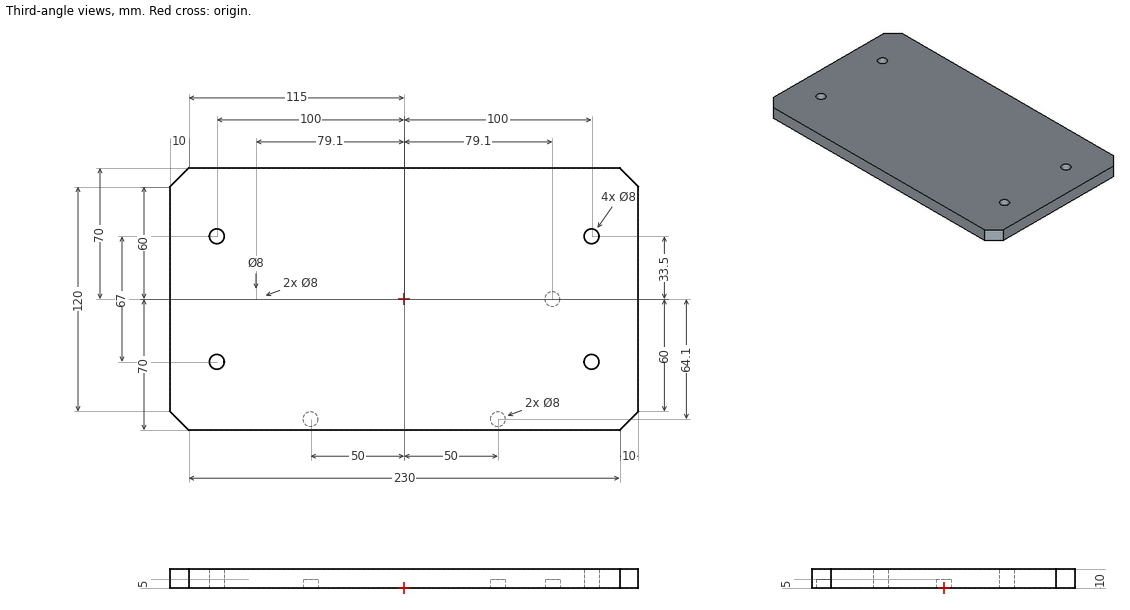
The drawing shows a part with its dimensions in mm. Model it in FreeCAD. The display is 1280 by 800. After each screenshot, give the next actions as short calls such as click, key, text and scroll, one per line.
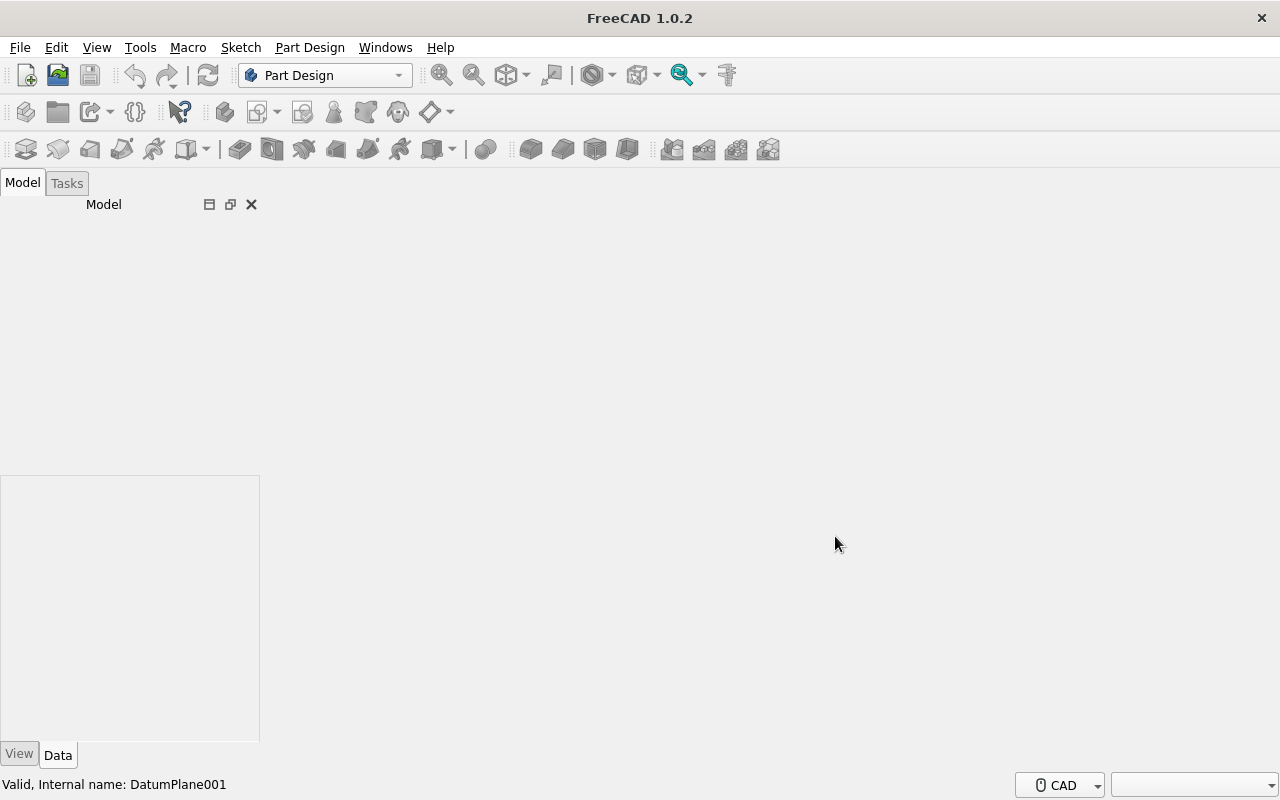
click(26, 76)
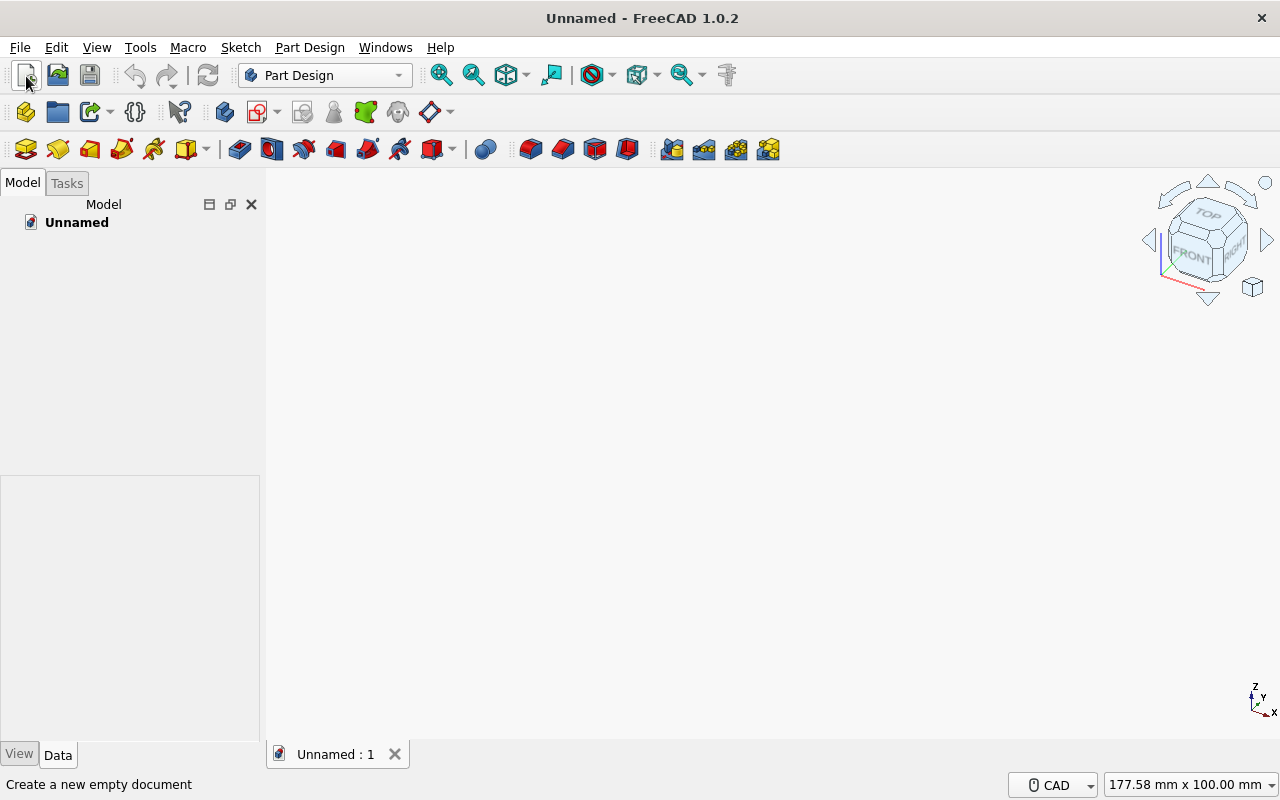
click(258, 112)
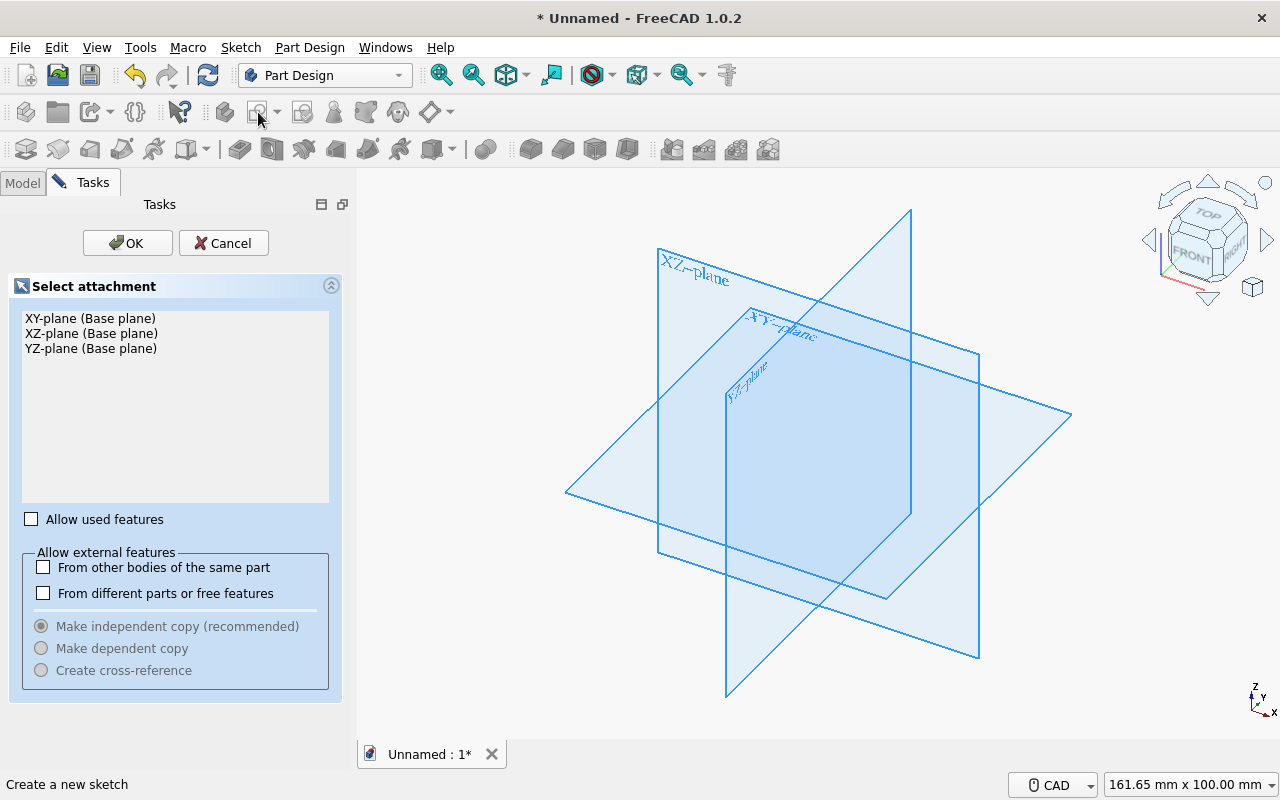
click(82, 318)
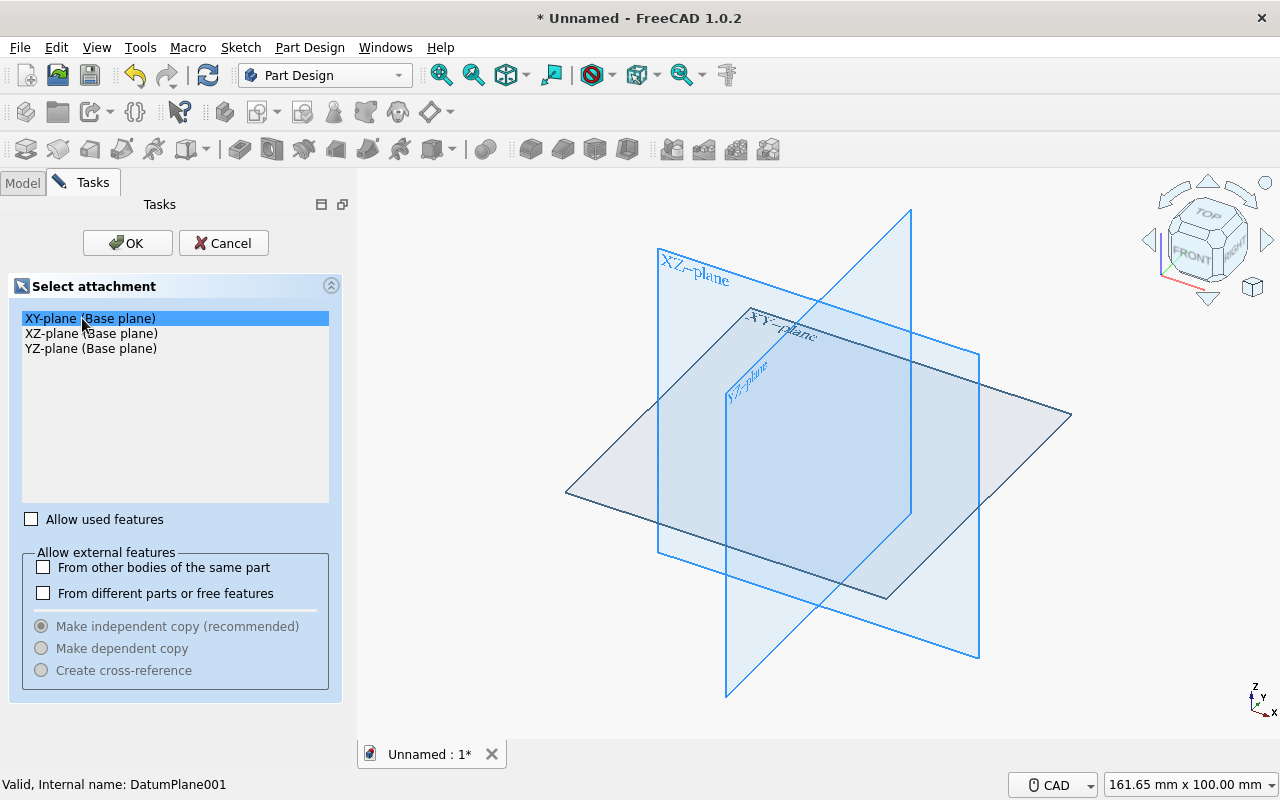
click(128, 243)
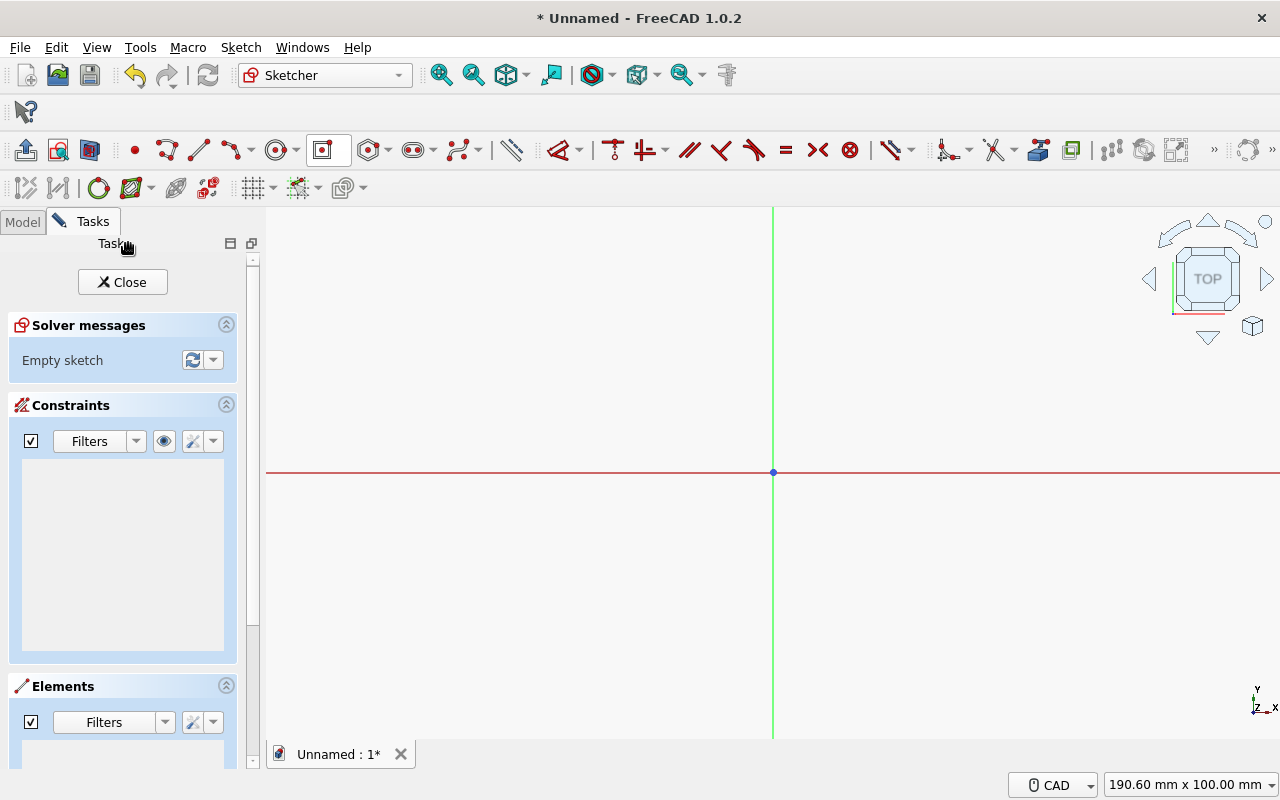
scroll(649, 473, down, 4)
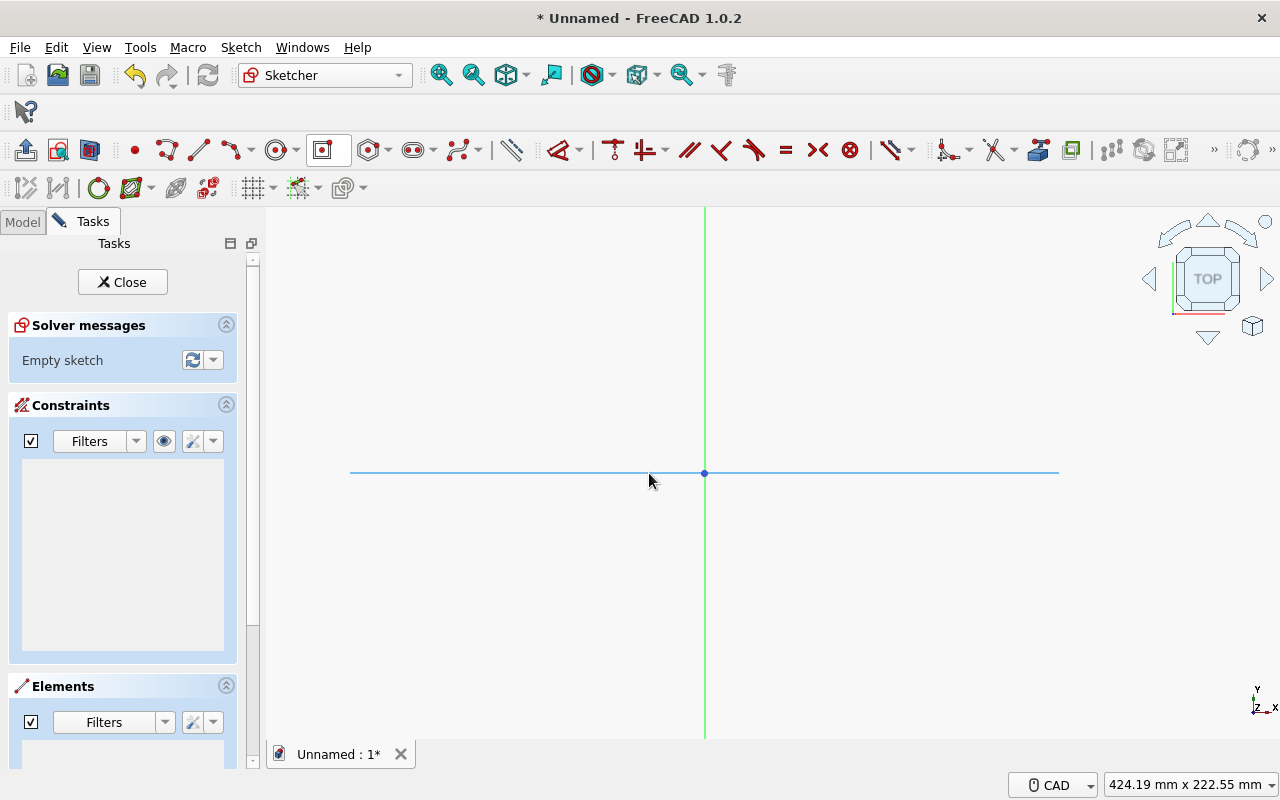
click(168, 150)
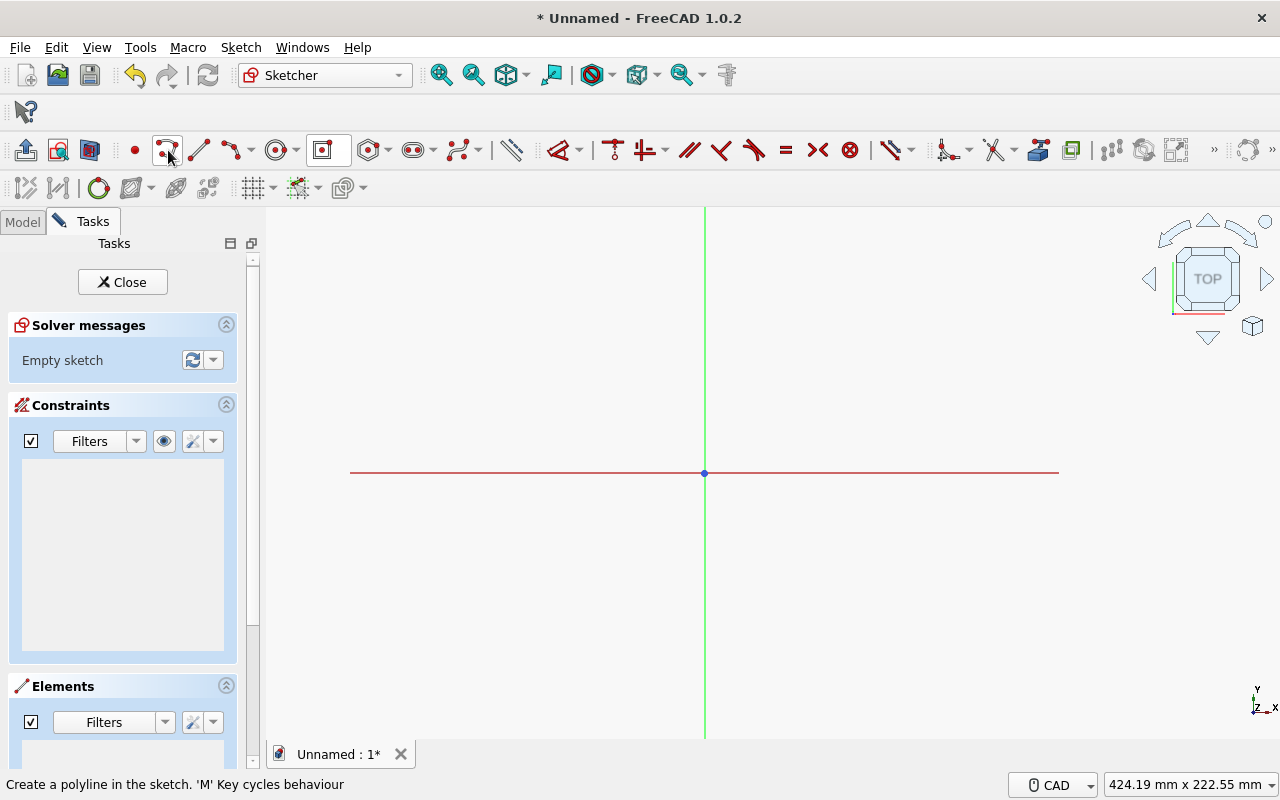
click(430, 306)
click(406, 330)
click(406, 617)
click(430, 641)
click(980, 641)
click(1004, 617)
click(1004, 330)
click(980, 306)
click(430, 307)
key(Escape)
key(Escape)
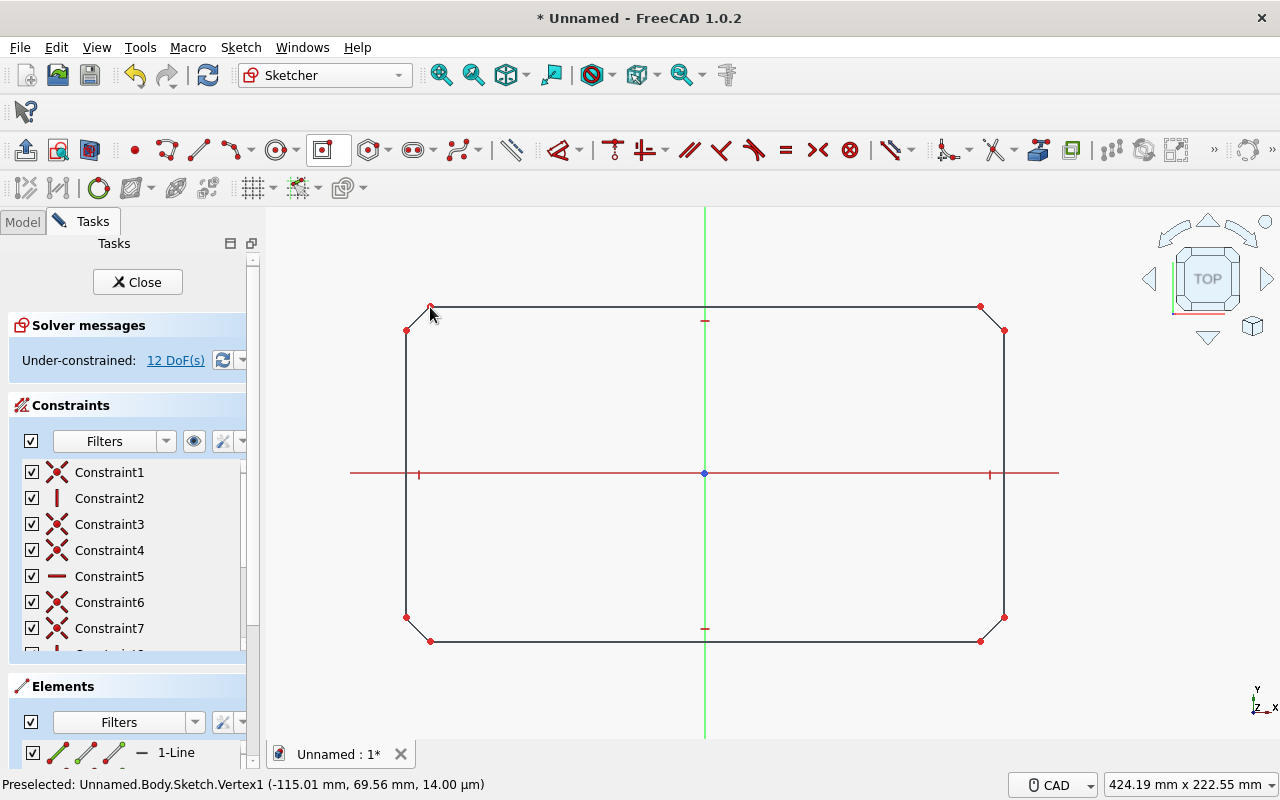
click(558, 150)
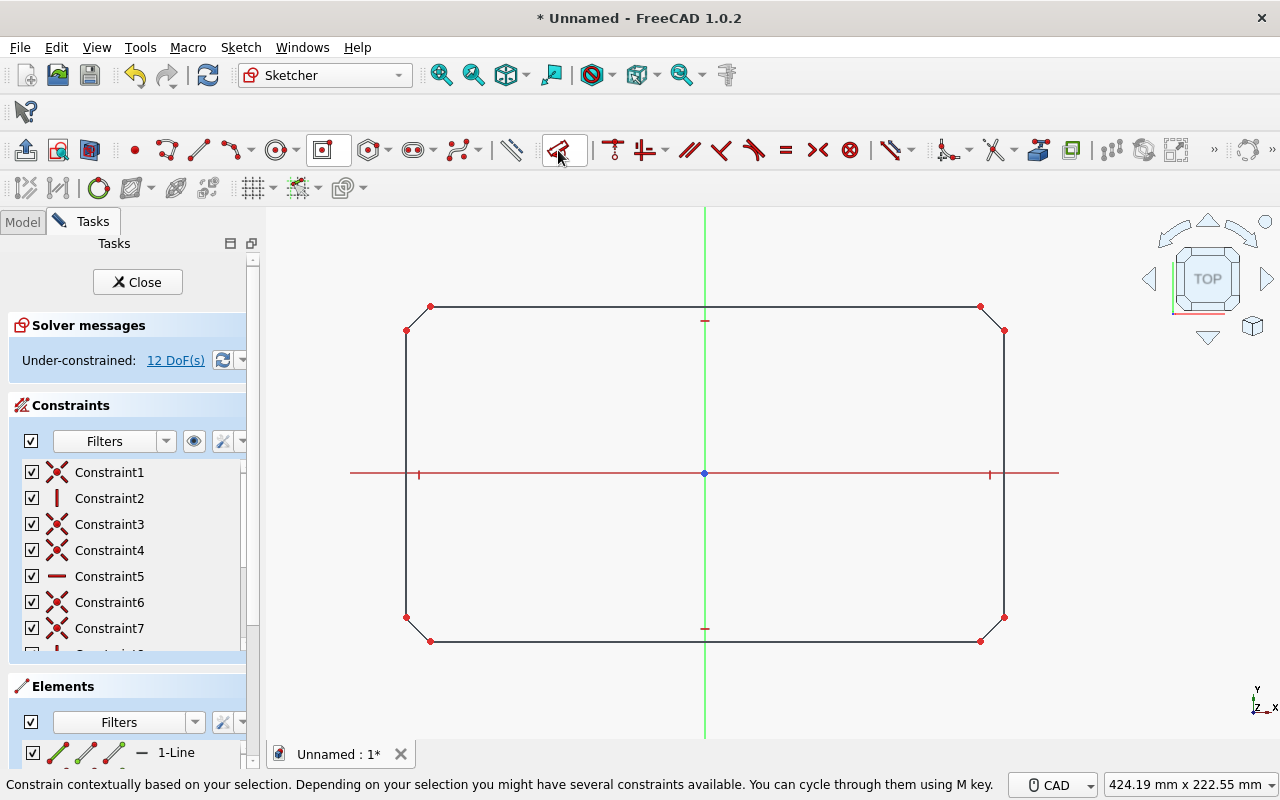
click(406, 417)
click(372, 408)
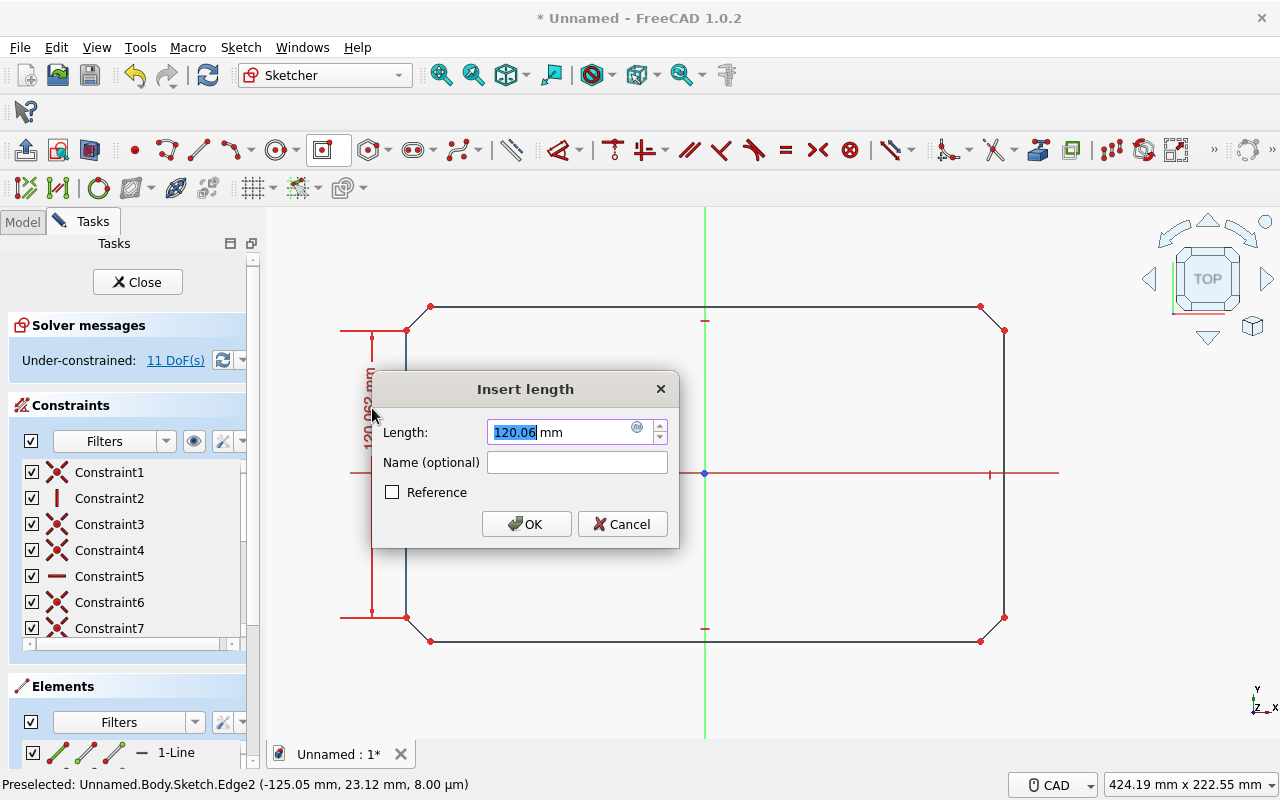
text(120)
key(Return)